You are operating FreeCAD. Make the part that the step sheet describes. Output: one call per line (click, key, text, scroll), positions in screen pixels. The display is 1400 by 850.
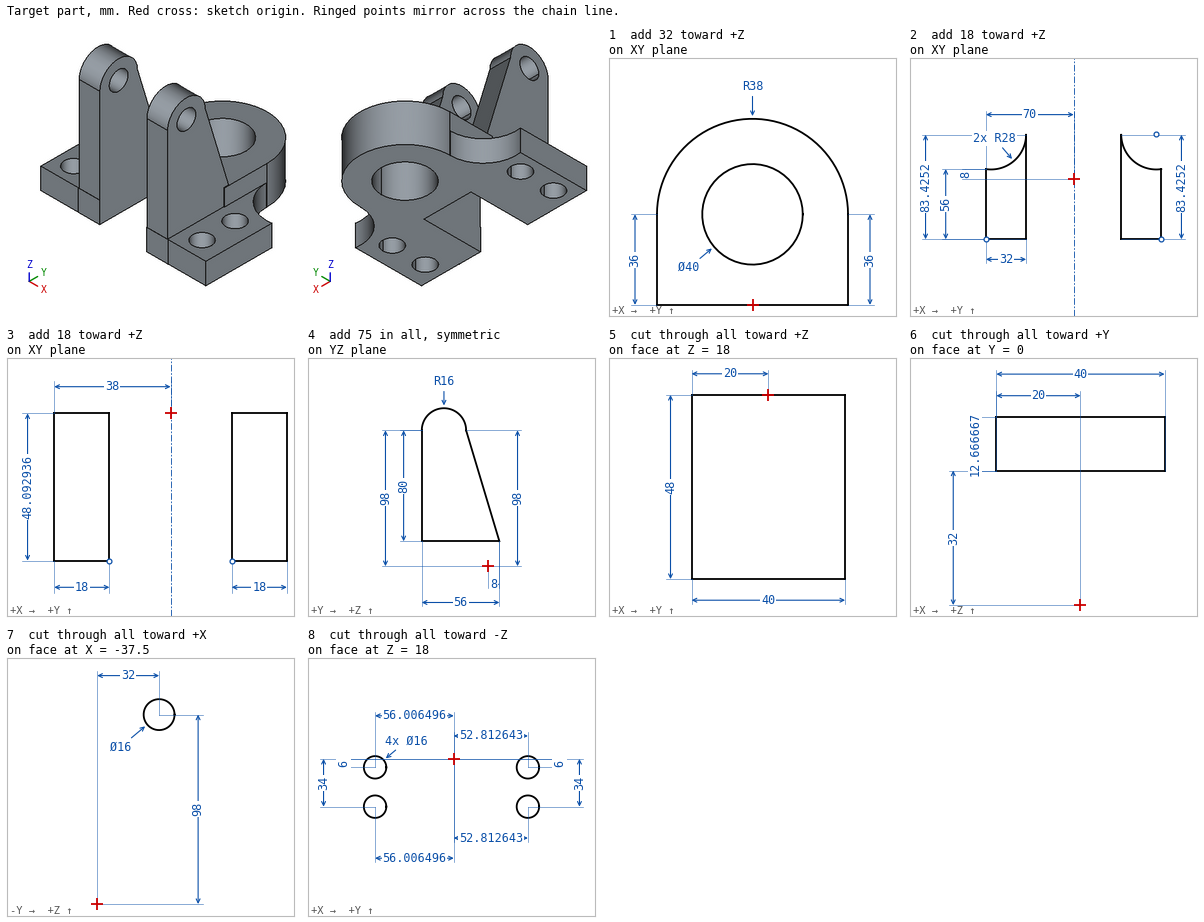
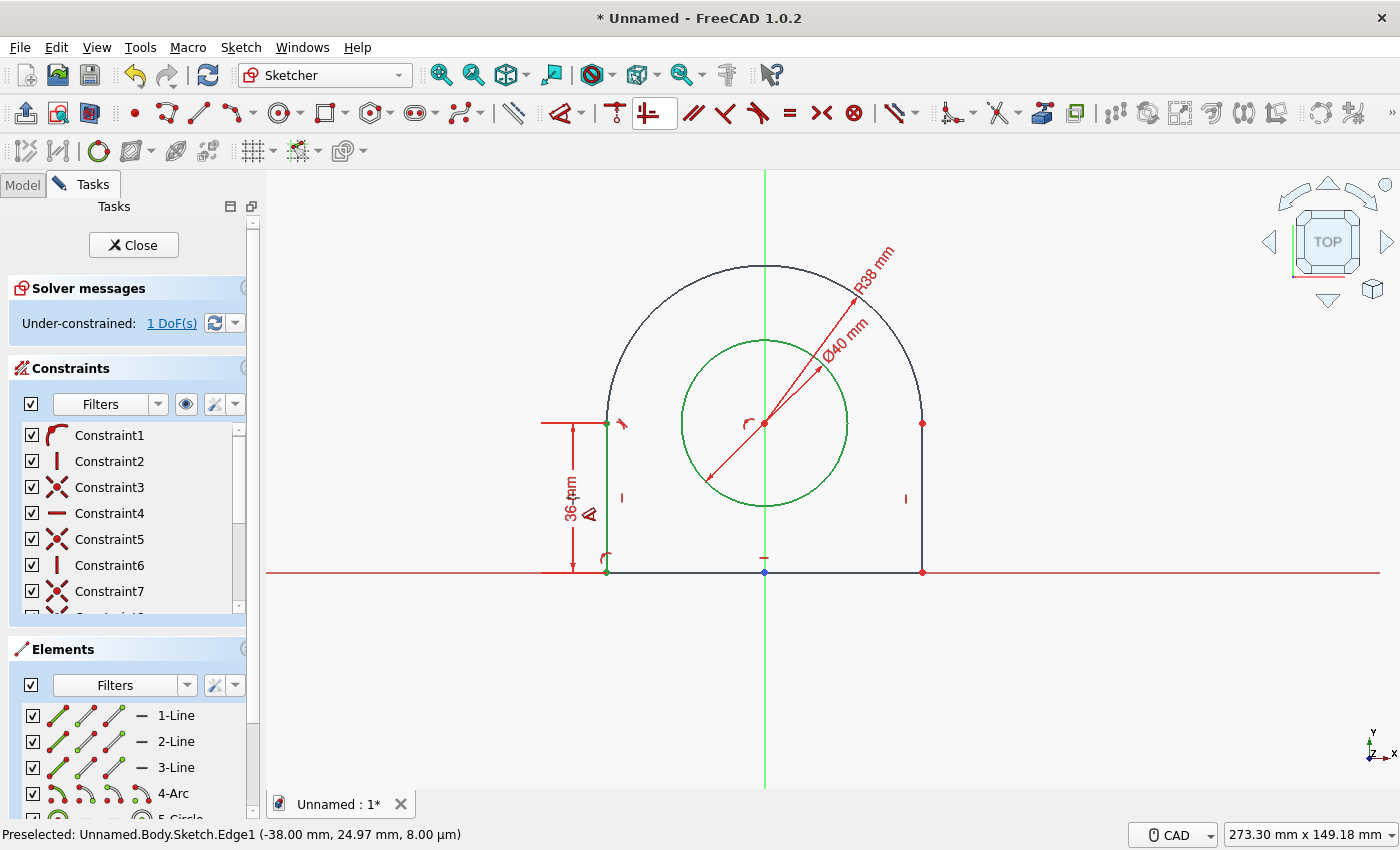
click(922, 528)
click(956, 498)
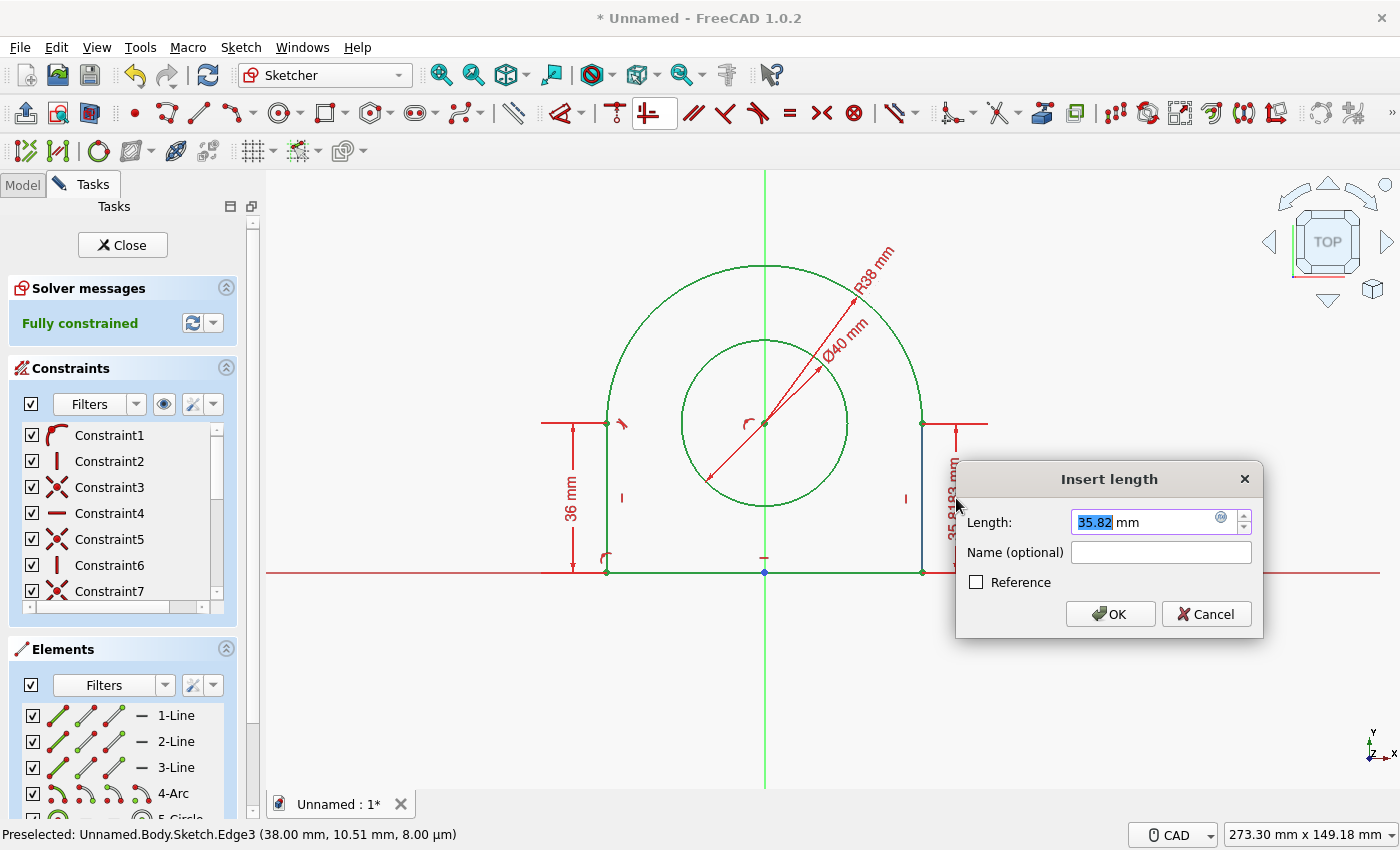
text(36)
key(Return)
key(Escape)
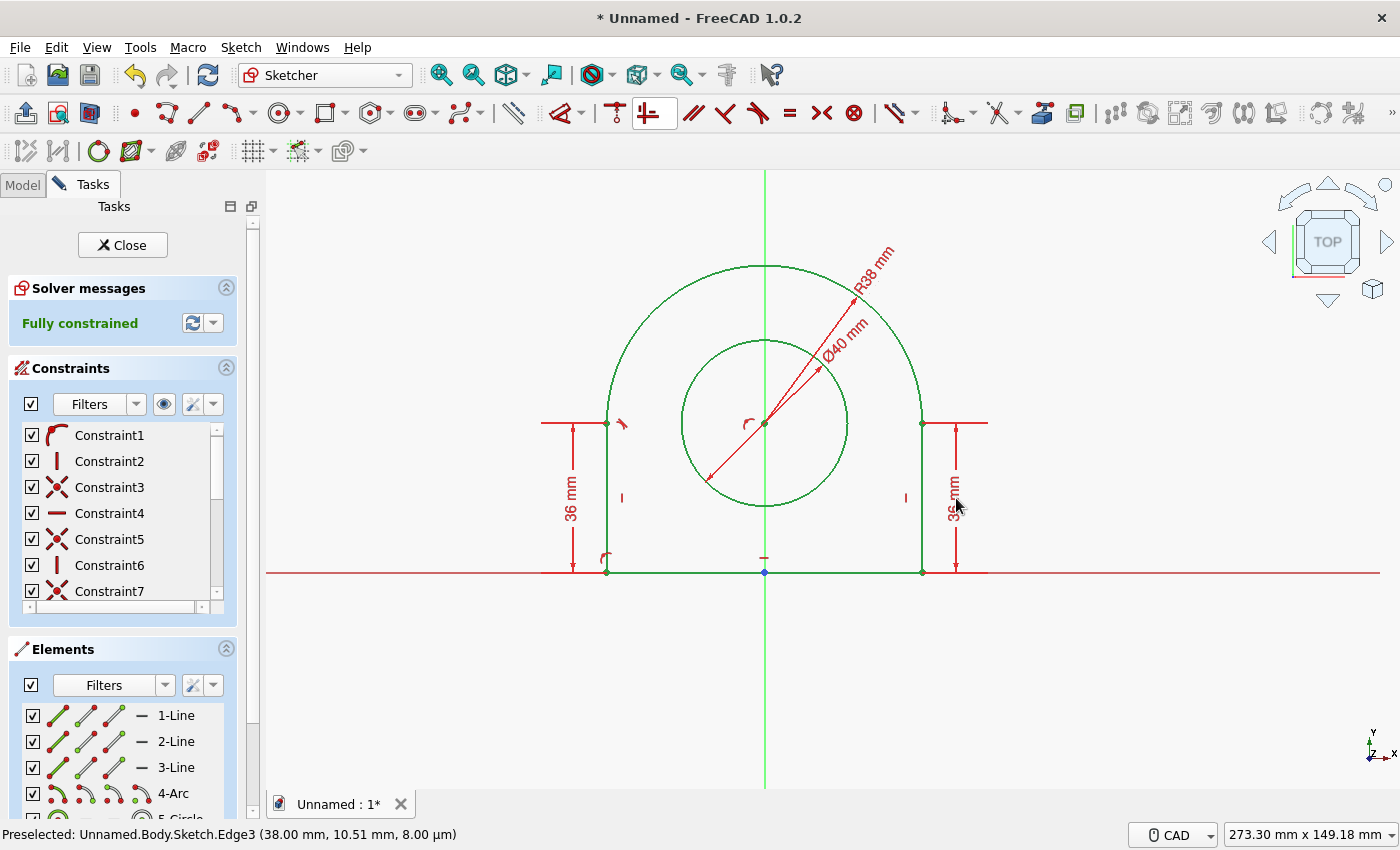
click(123, 245)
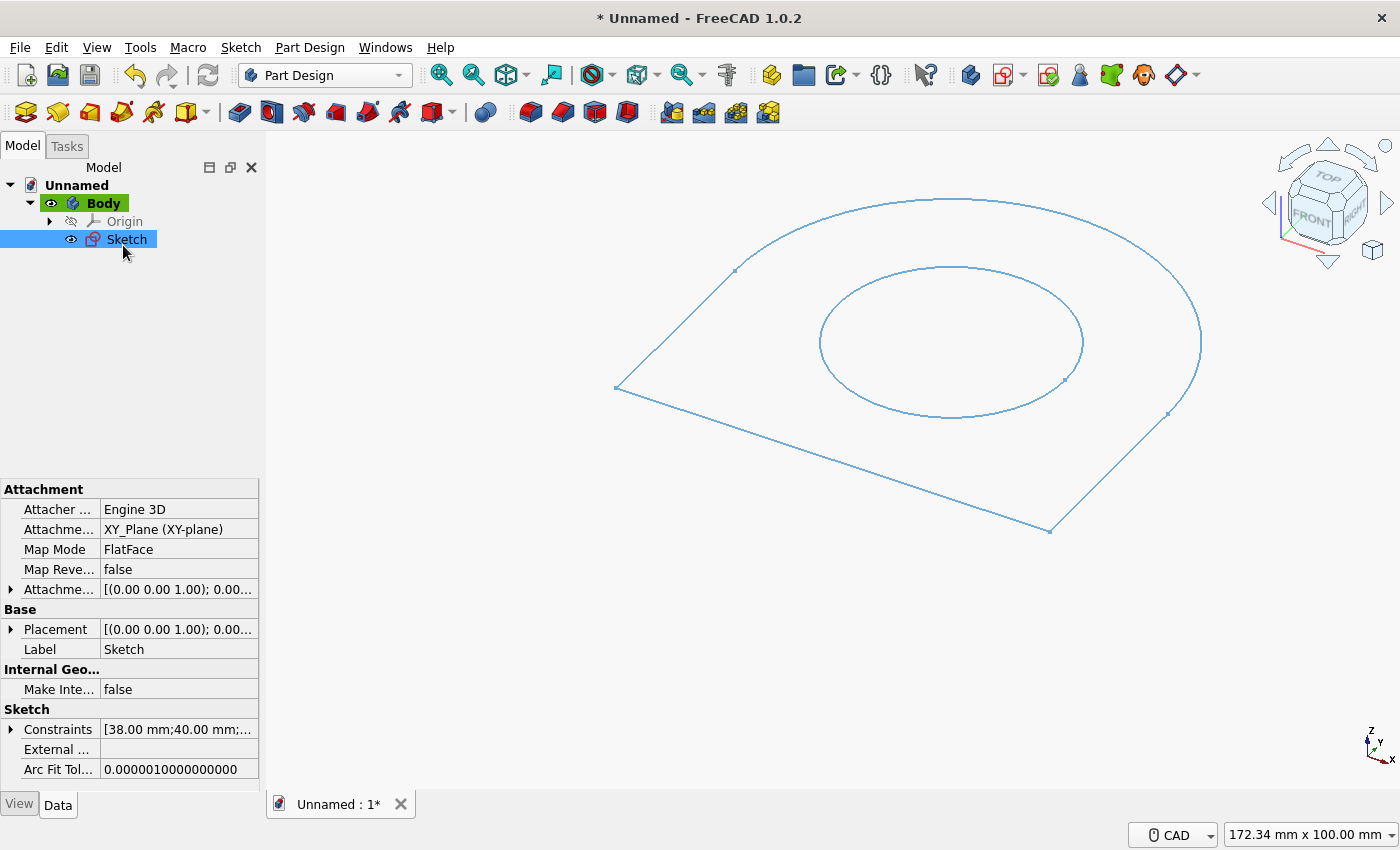
click(26, 112)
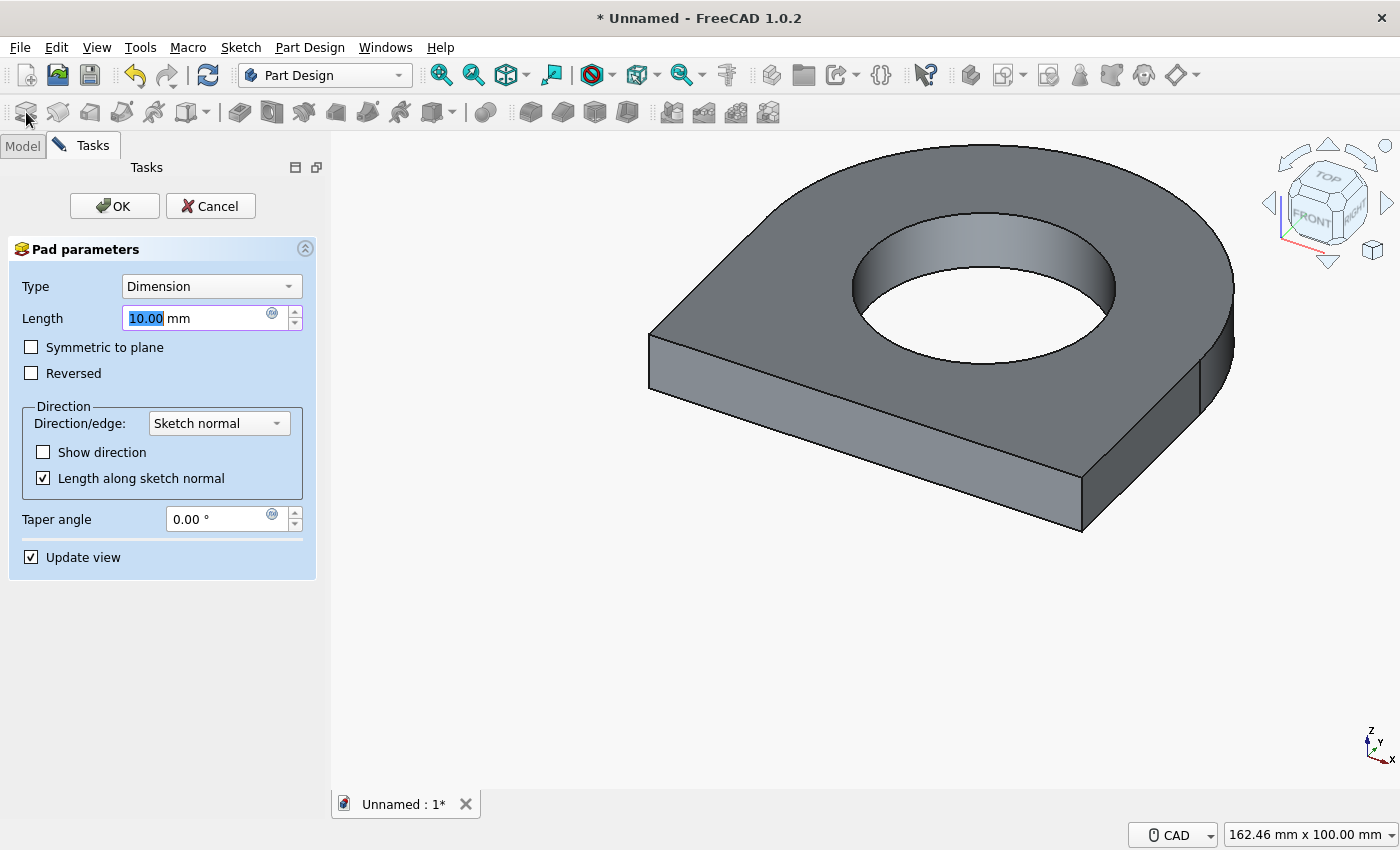
text(32)
key(Tab)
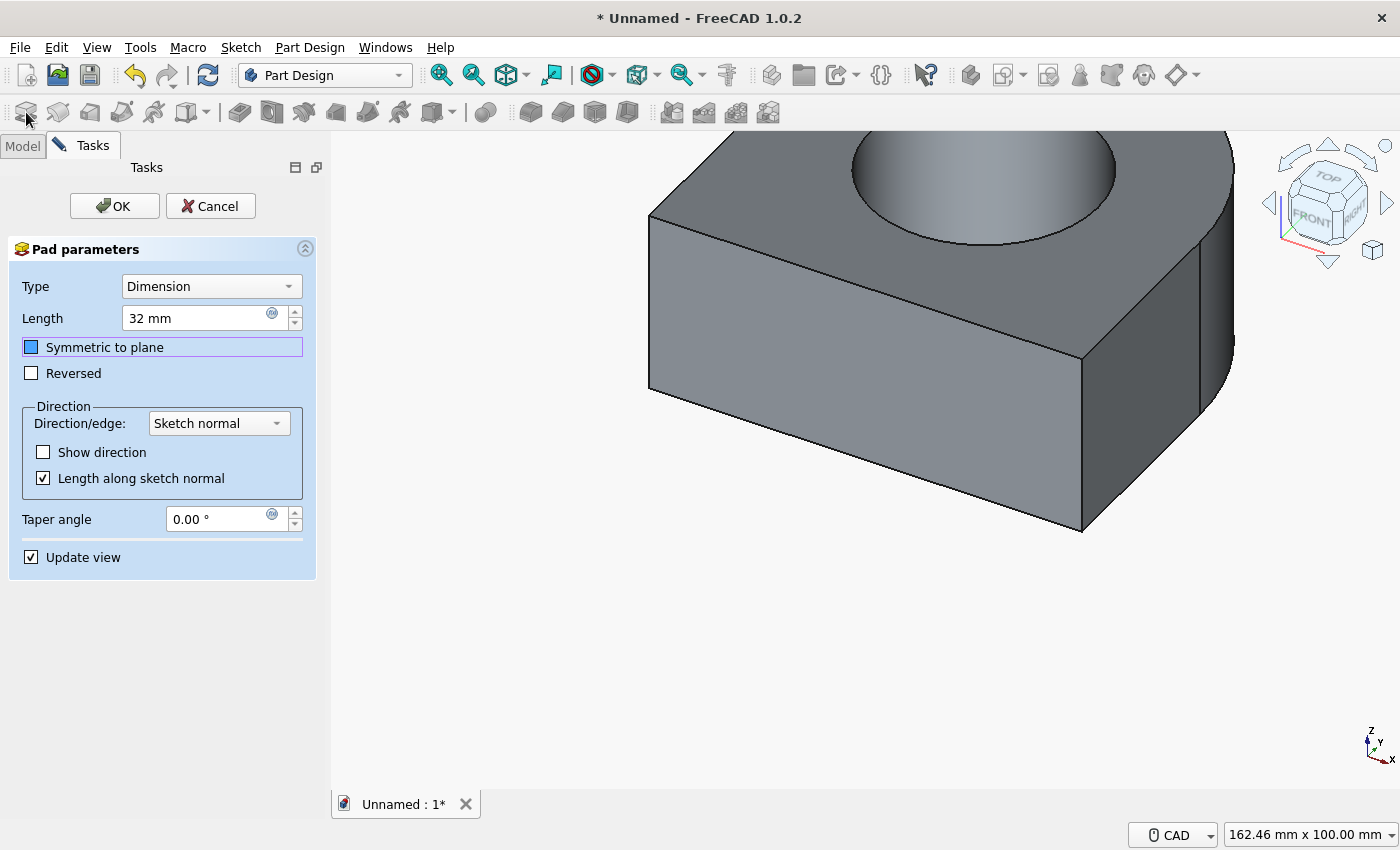
click(115, 206)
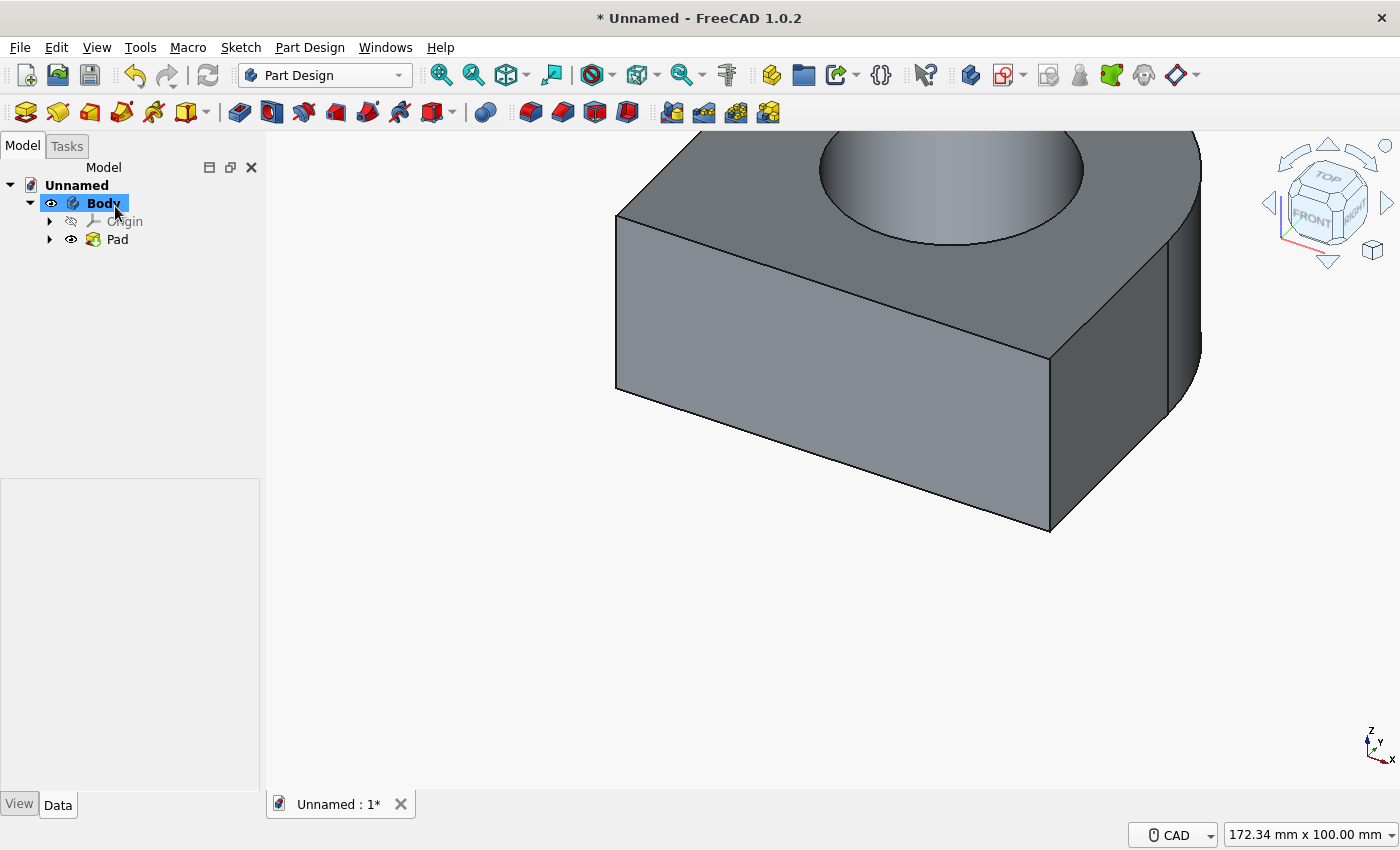
click(442, 76)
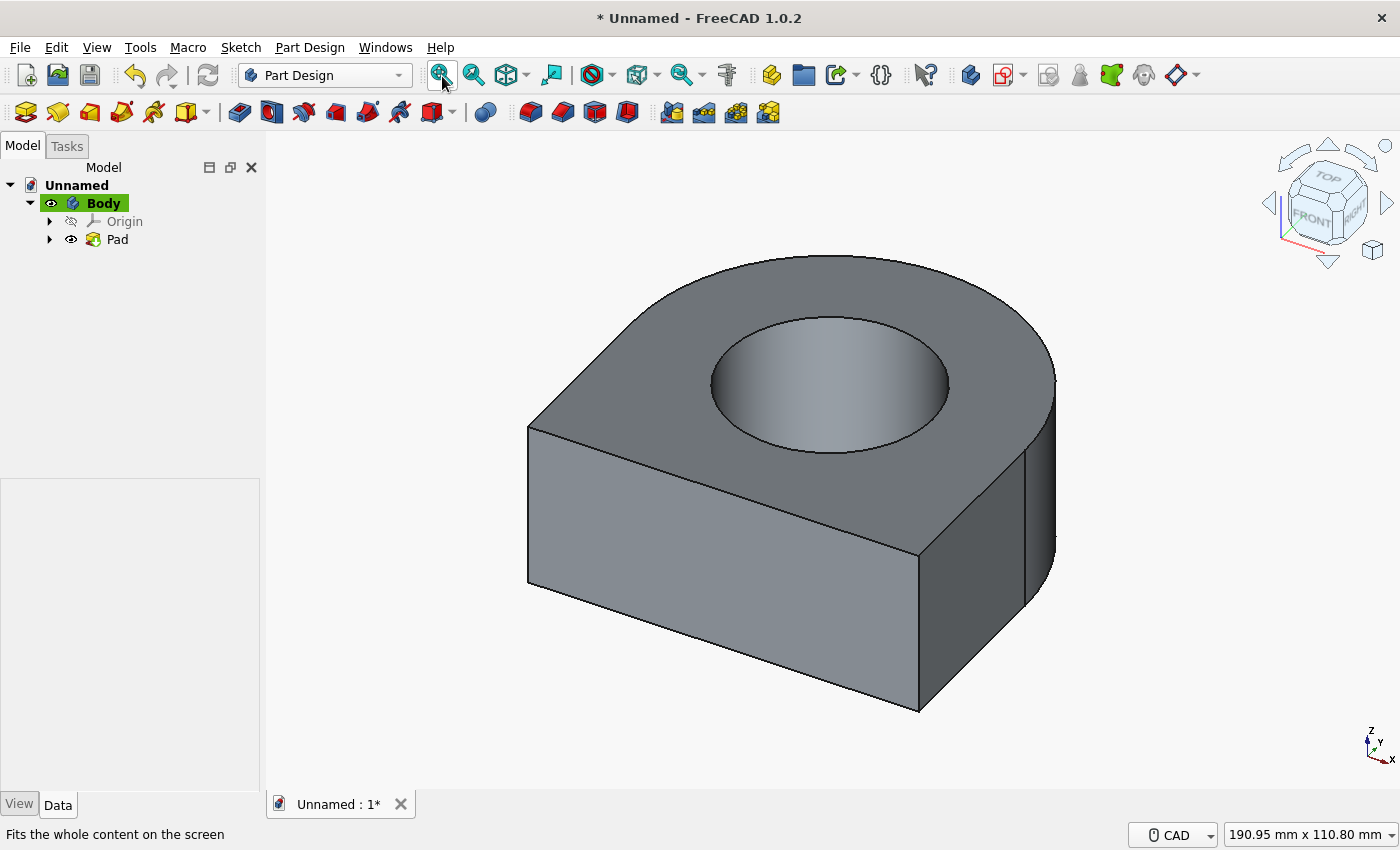
click(1004, 76)